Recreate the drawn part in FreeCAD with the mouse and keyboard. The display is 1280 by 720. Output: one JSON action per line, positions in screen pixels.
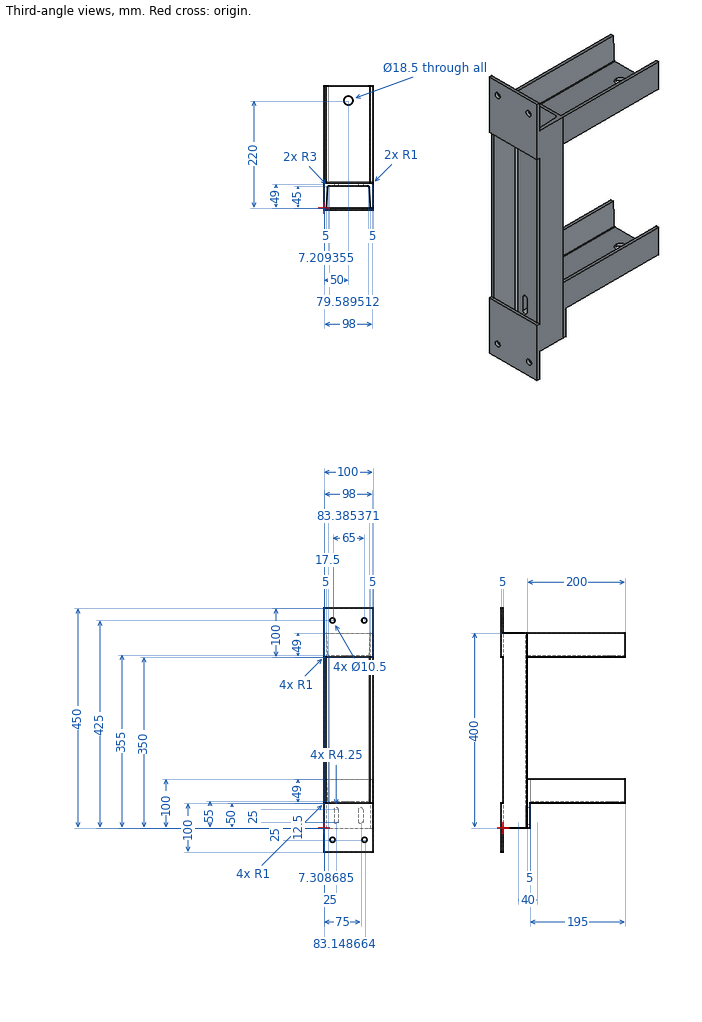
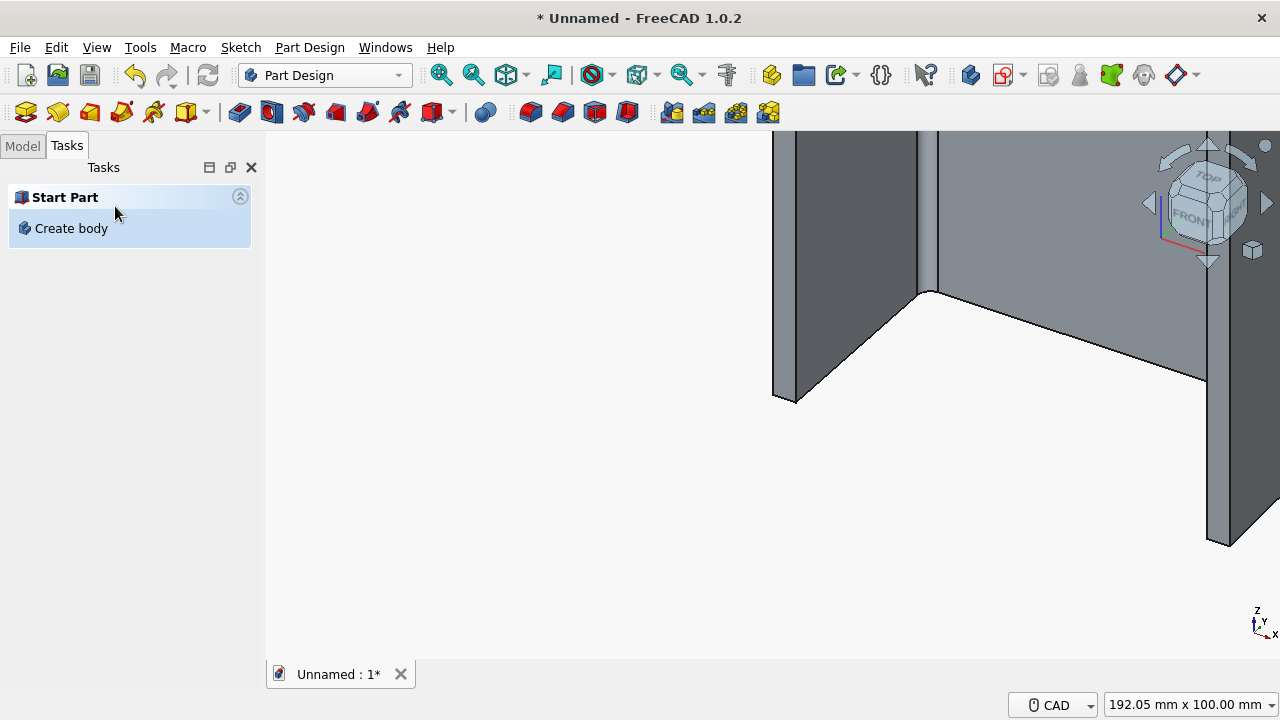
{"action": "left_click", "coordinate": [442, 76]}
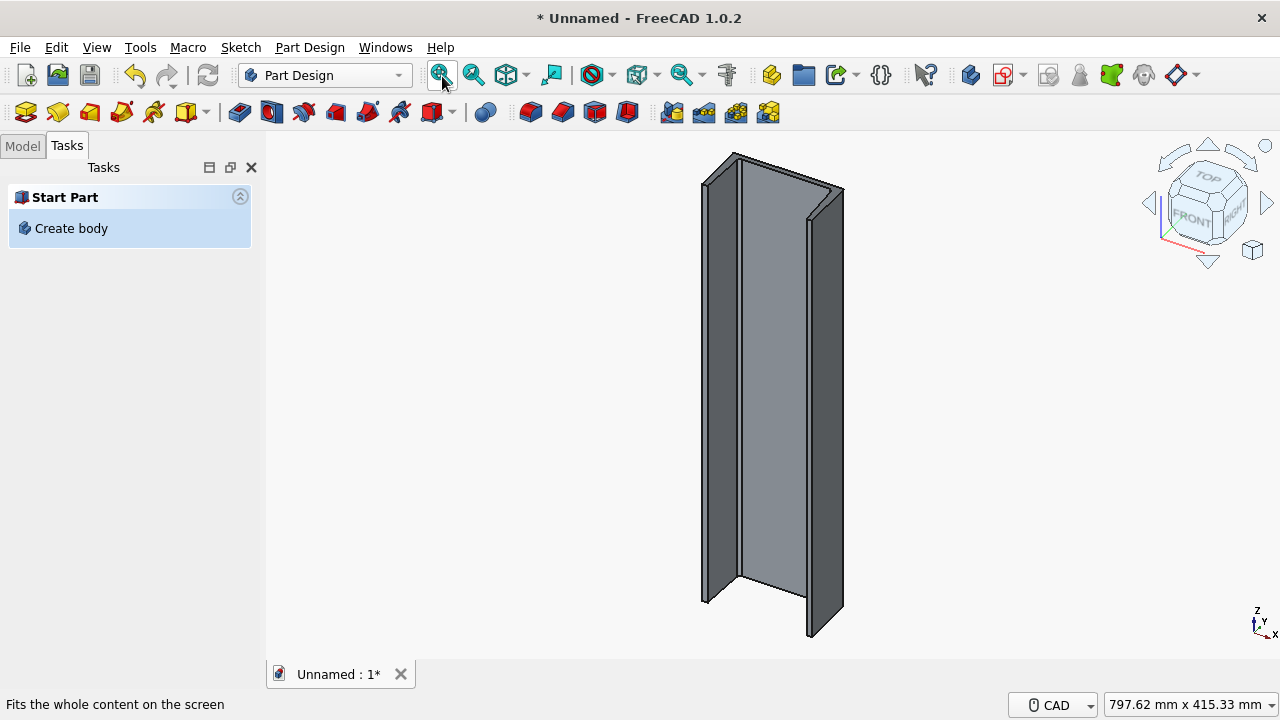
{"action": "left_click", "coordinate": [1004, 76]}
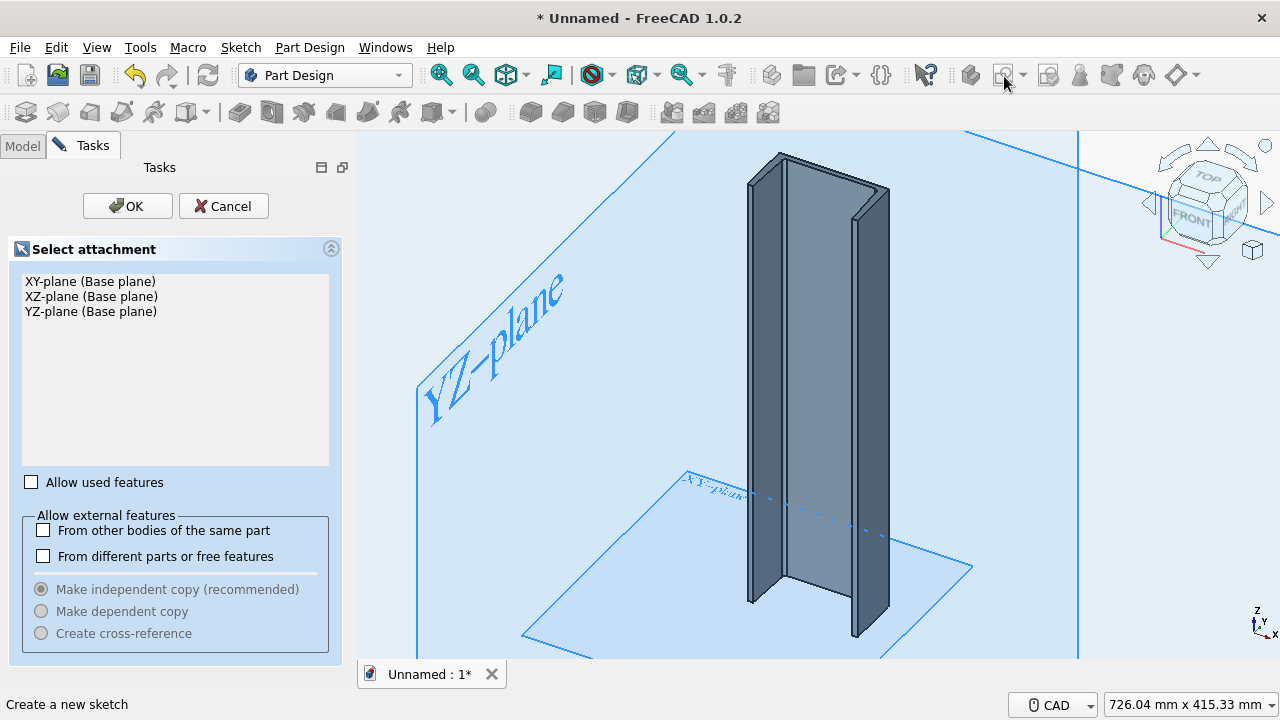
{"action": "left_click", "coordinate": [82, 296]}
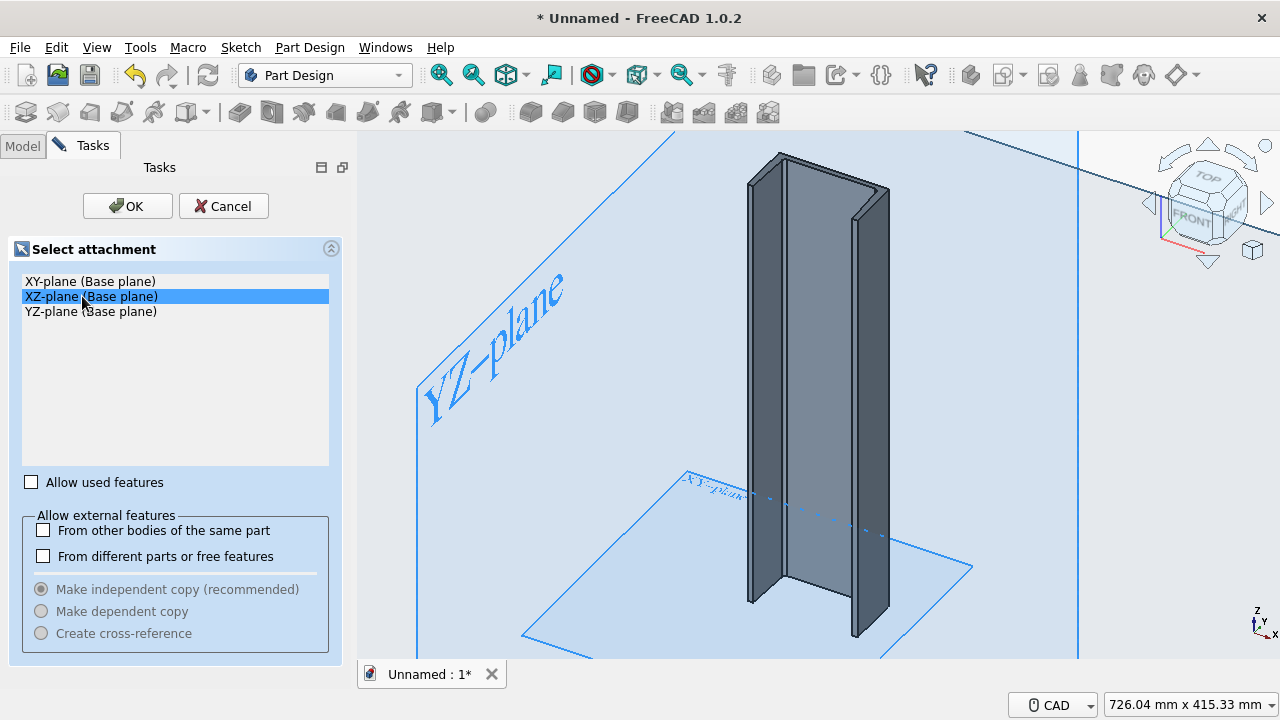
{"action": "left_click", "coordinate": [128, 206]}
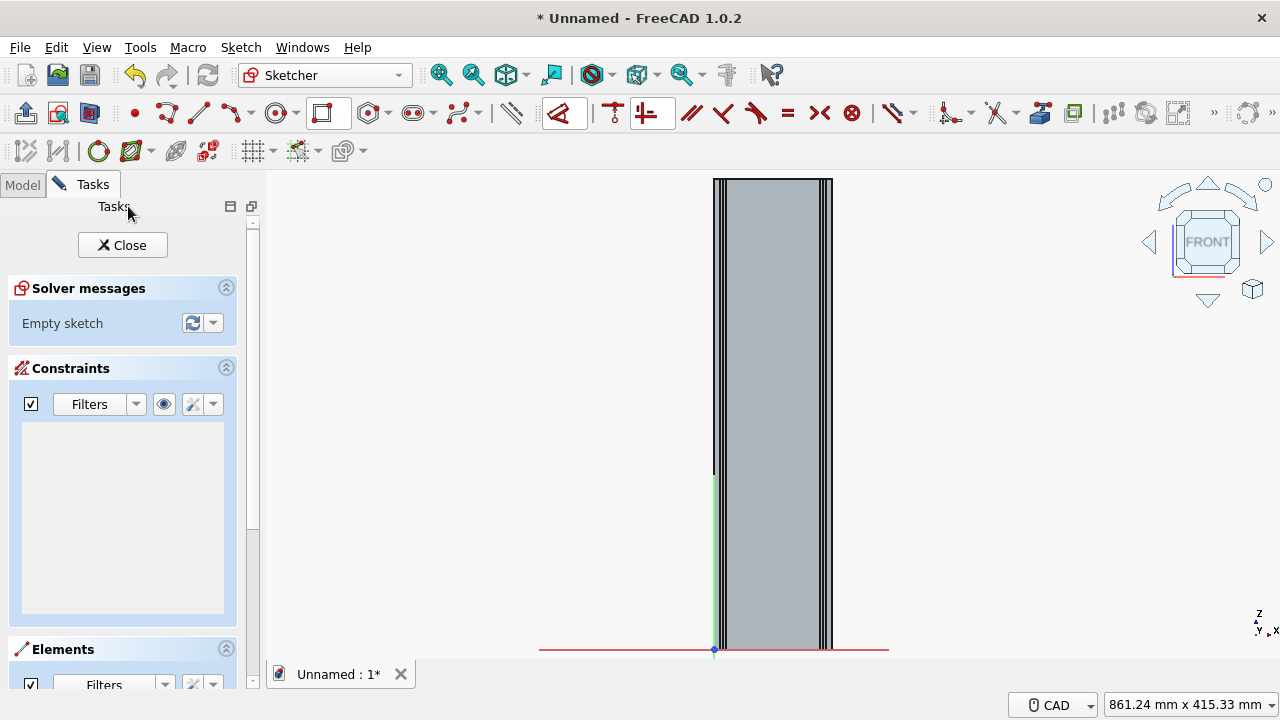
{"action": "scroll", "coordinate": [621, 414], "scroll_direction": "down", "scroll_amount": 3}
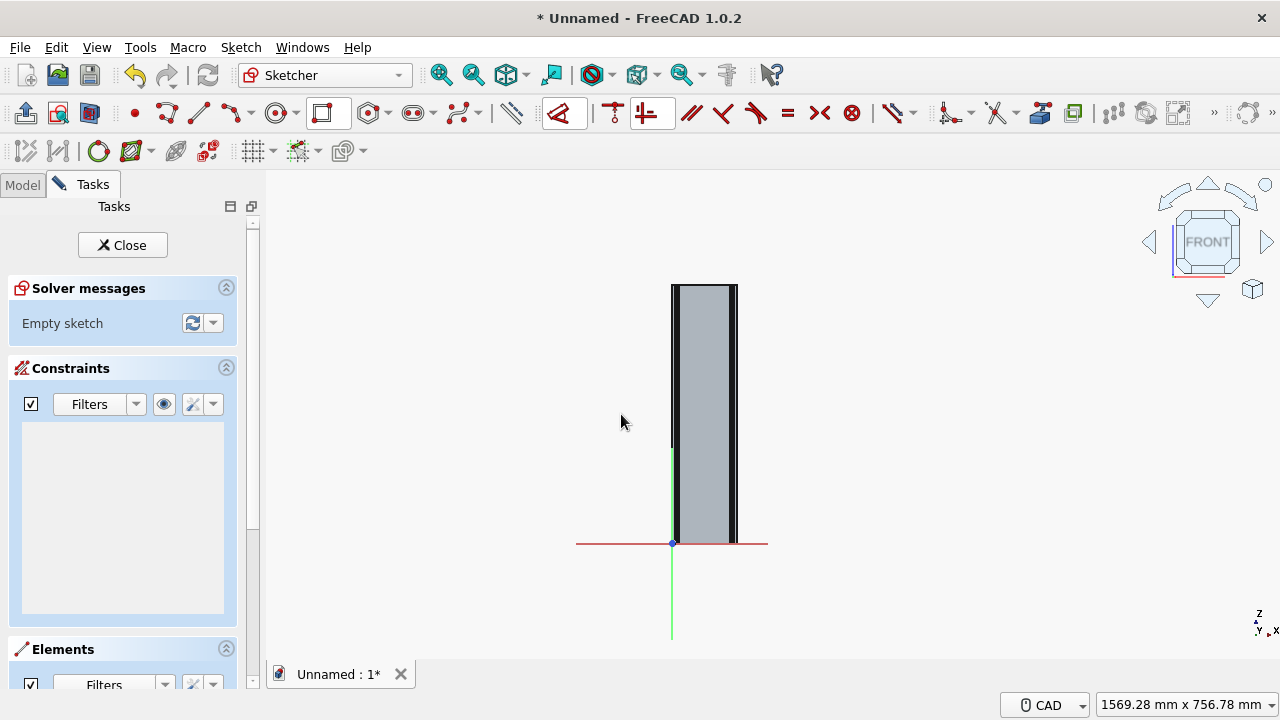
{"action": "left_click", "coordinate": [322, 114]}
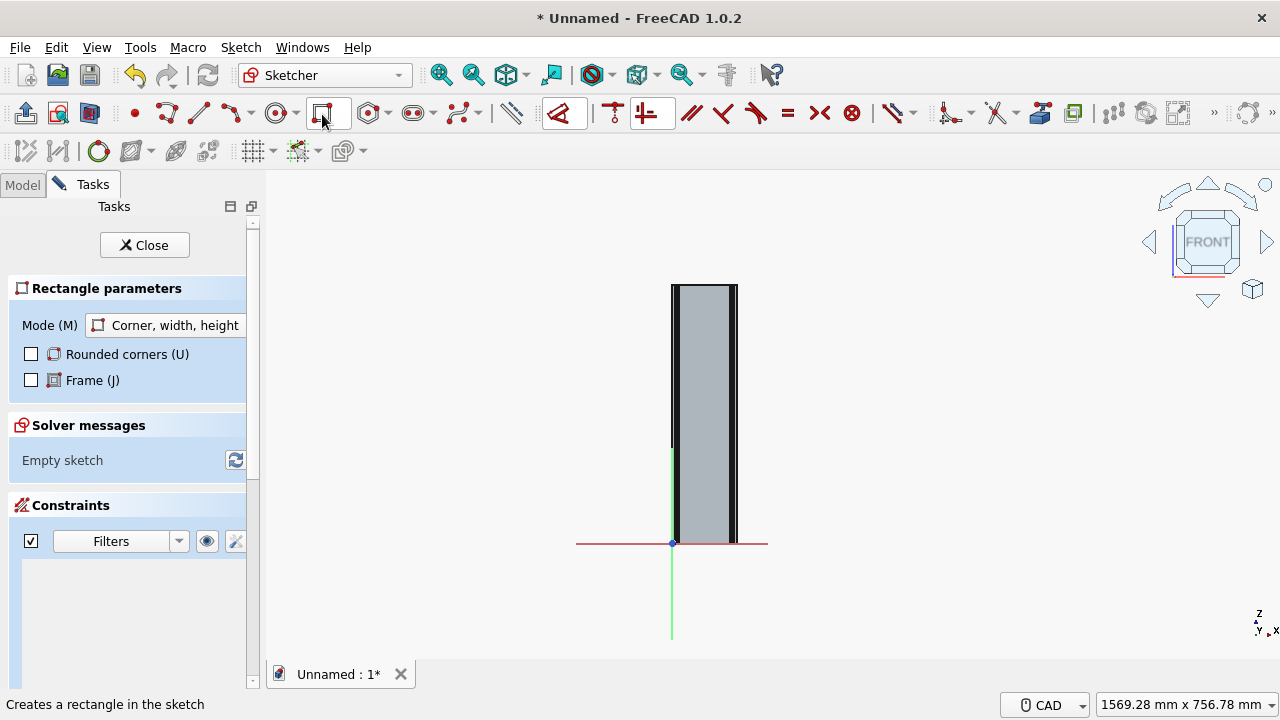
{"action": "left_click", "coordinate": [672, 253]}
{"action": "left_click", "coordinate": [737, 318]}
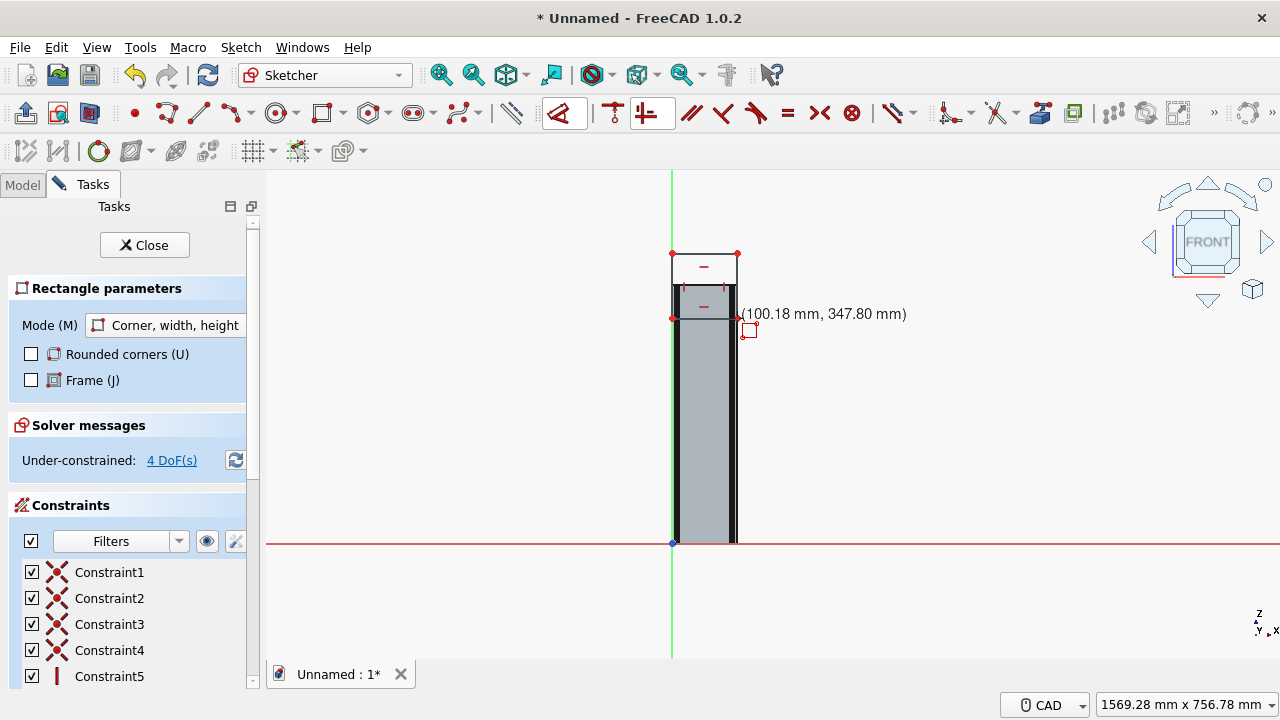
{"action": "left_click", "coordinate": [672, 511]}
{"action": "left_click", "coordinate": [737, 576]}
{"action": "key", "text": "Escape"}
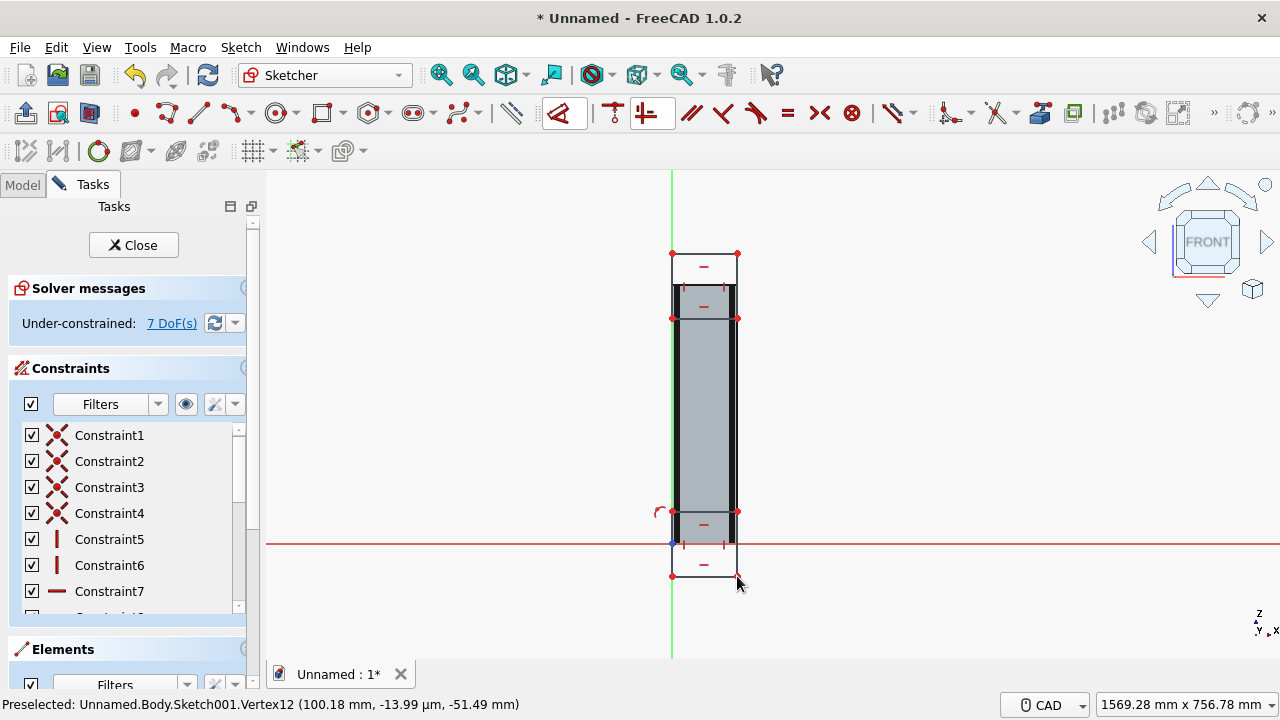
{"action": "left_click", "coordinate": [672, 254]}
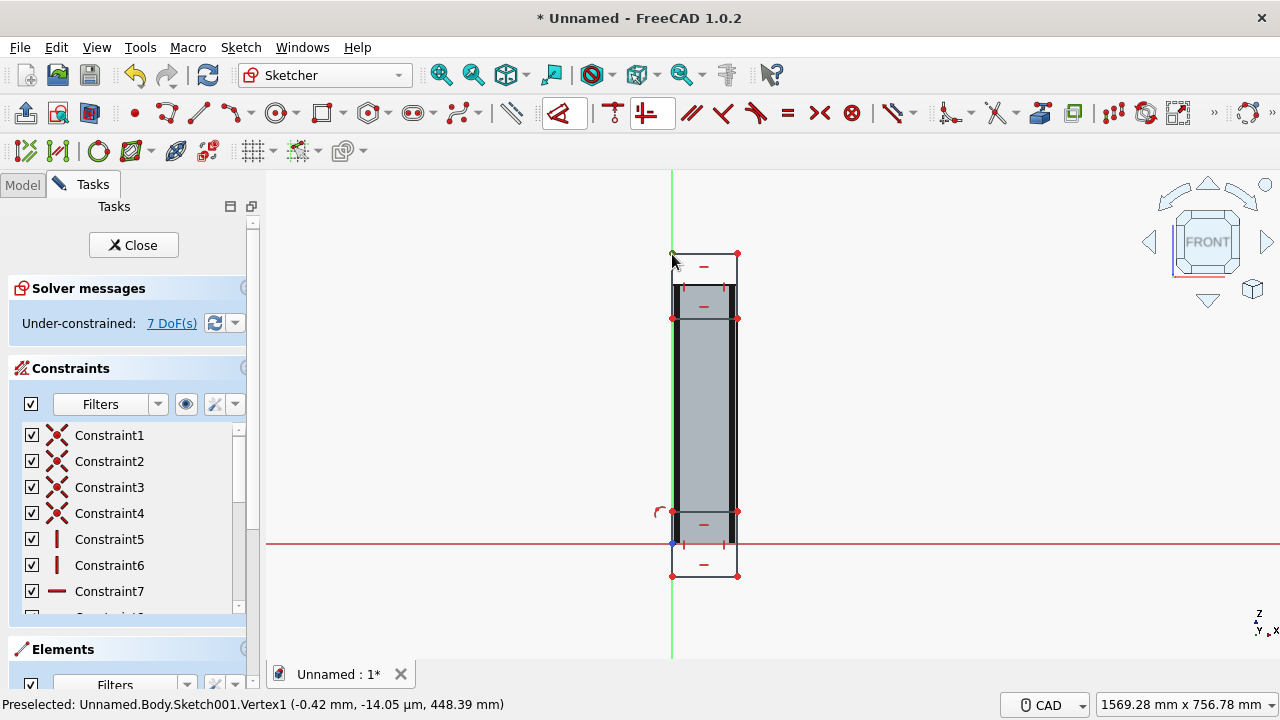
{"action": "left_click", "coordinate": [672, 476]}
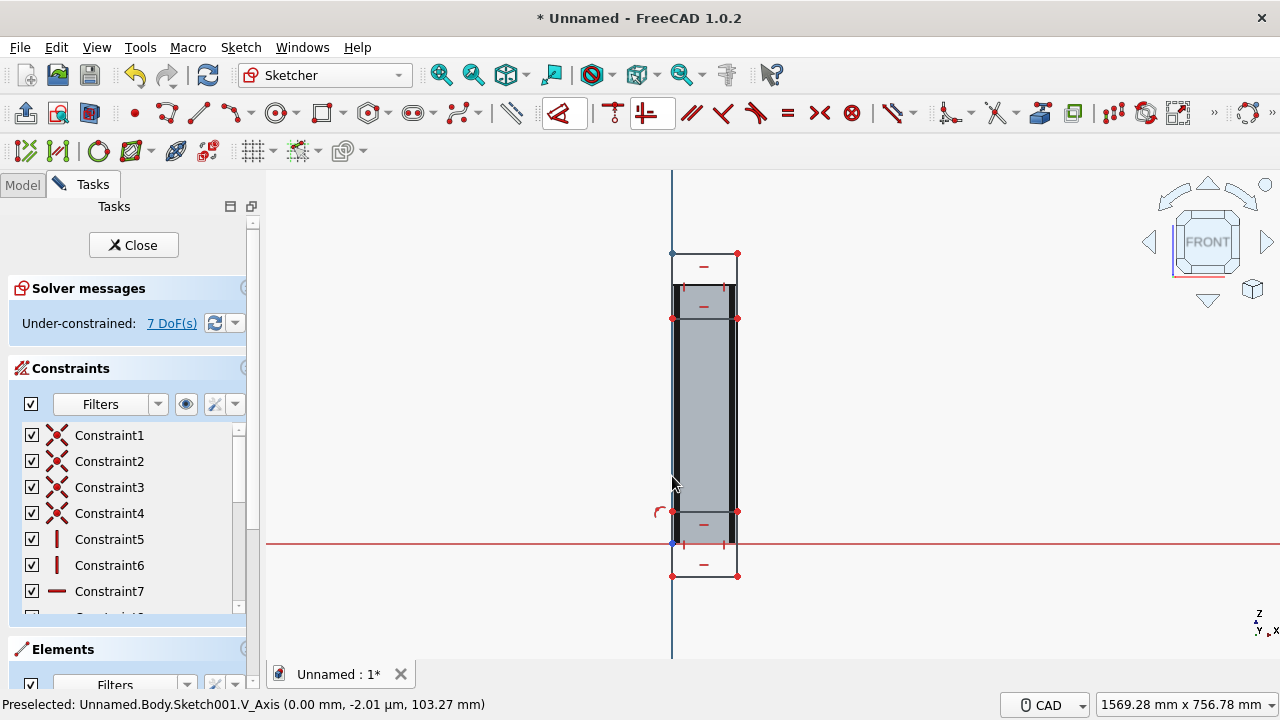
{"action": "left_click", "coordinate": [614, 114]}